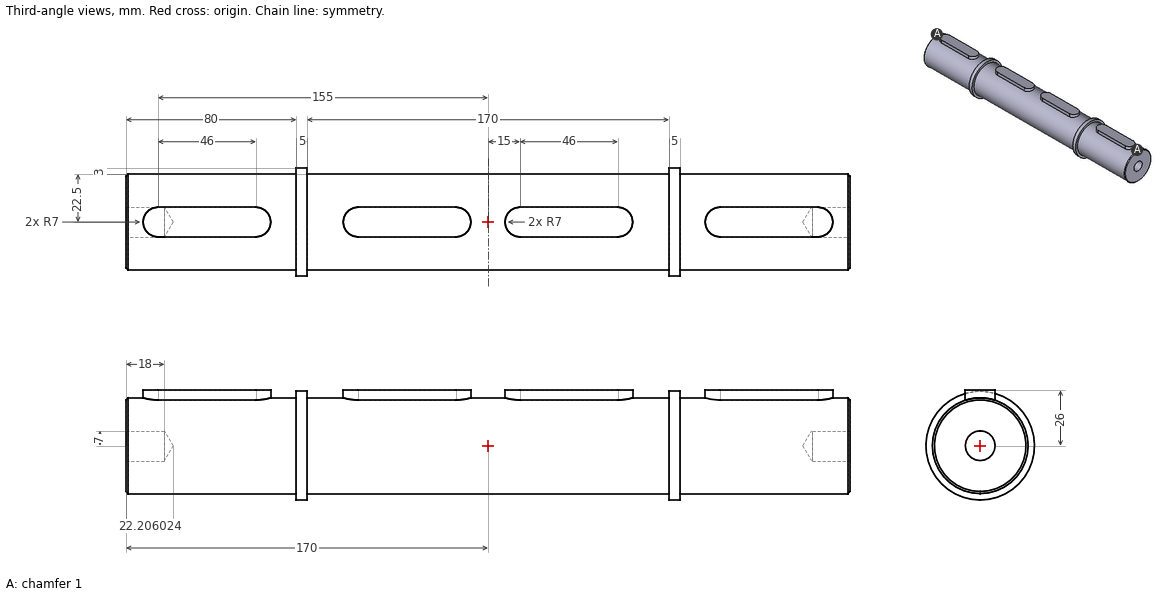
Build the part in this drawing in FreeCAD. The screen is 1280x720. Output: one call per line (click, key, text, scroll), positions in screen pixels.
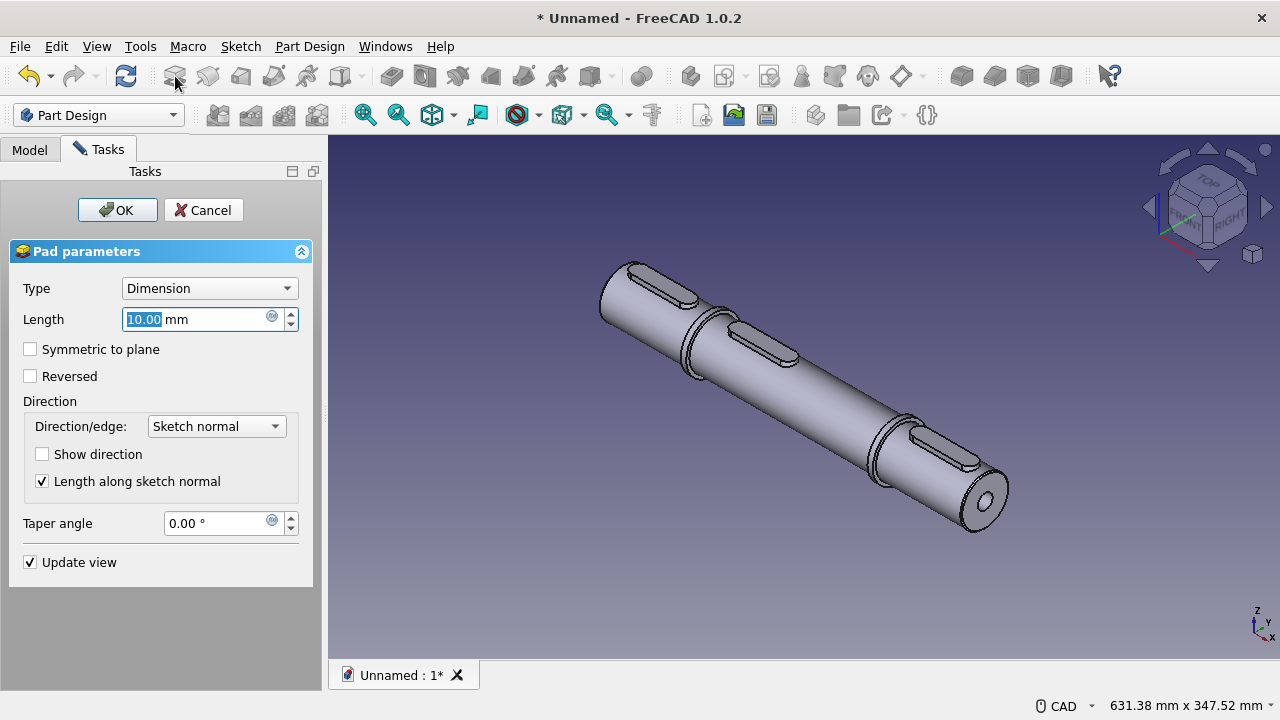
text(26)
key(Tab)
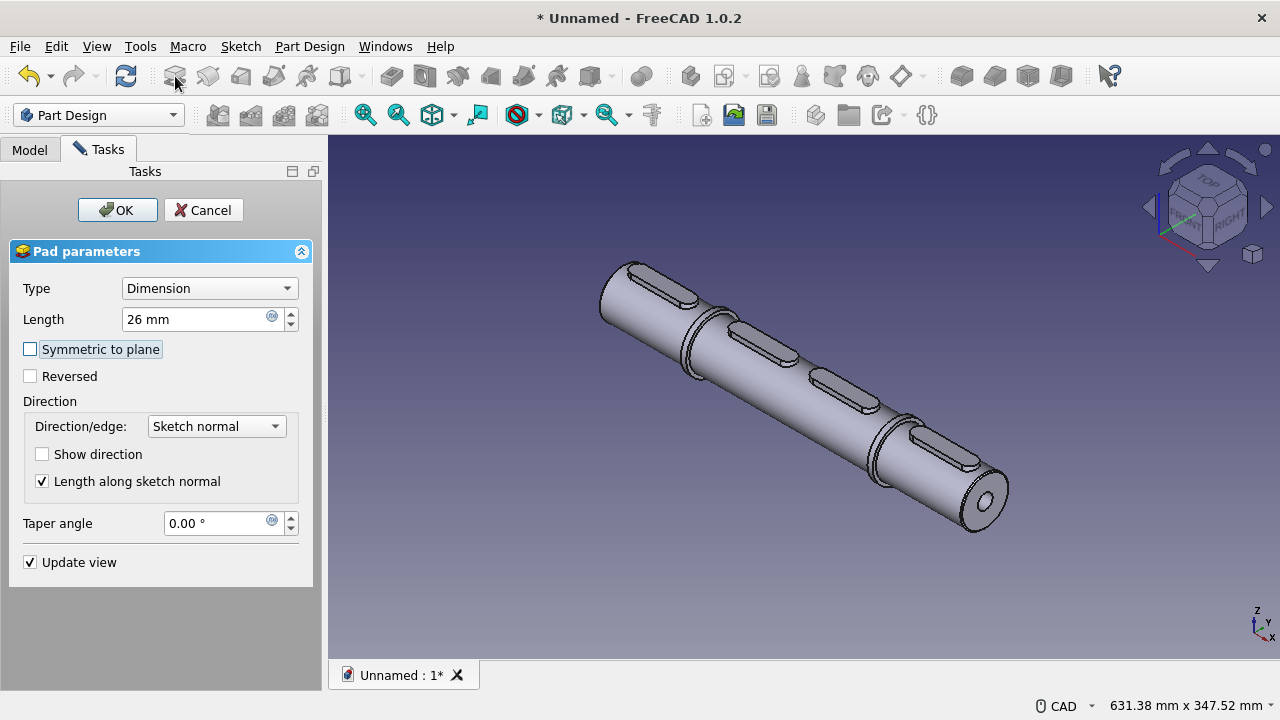
click(118, 210)